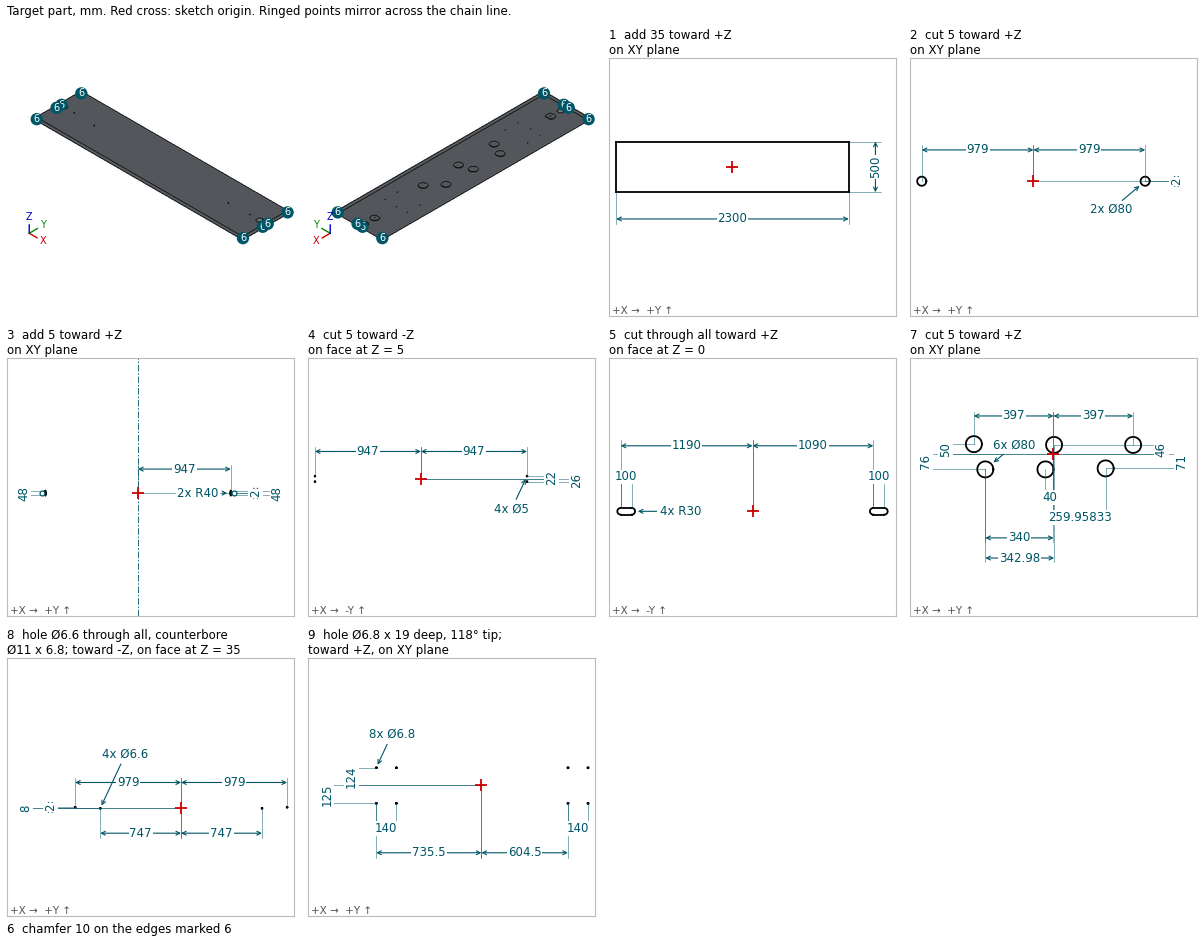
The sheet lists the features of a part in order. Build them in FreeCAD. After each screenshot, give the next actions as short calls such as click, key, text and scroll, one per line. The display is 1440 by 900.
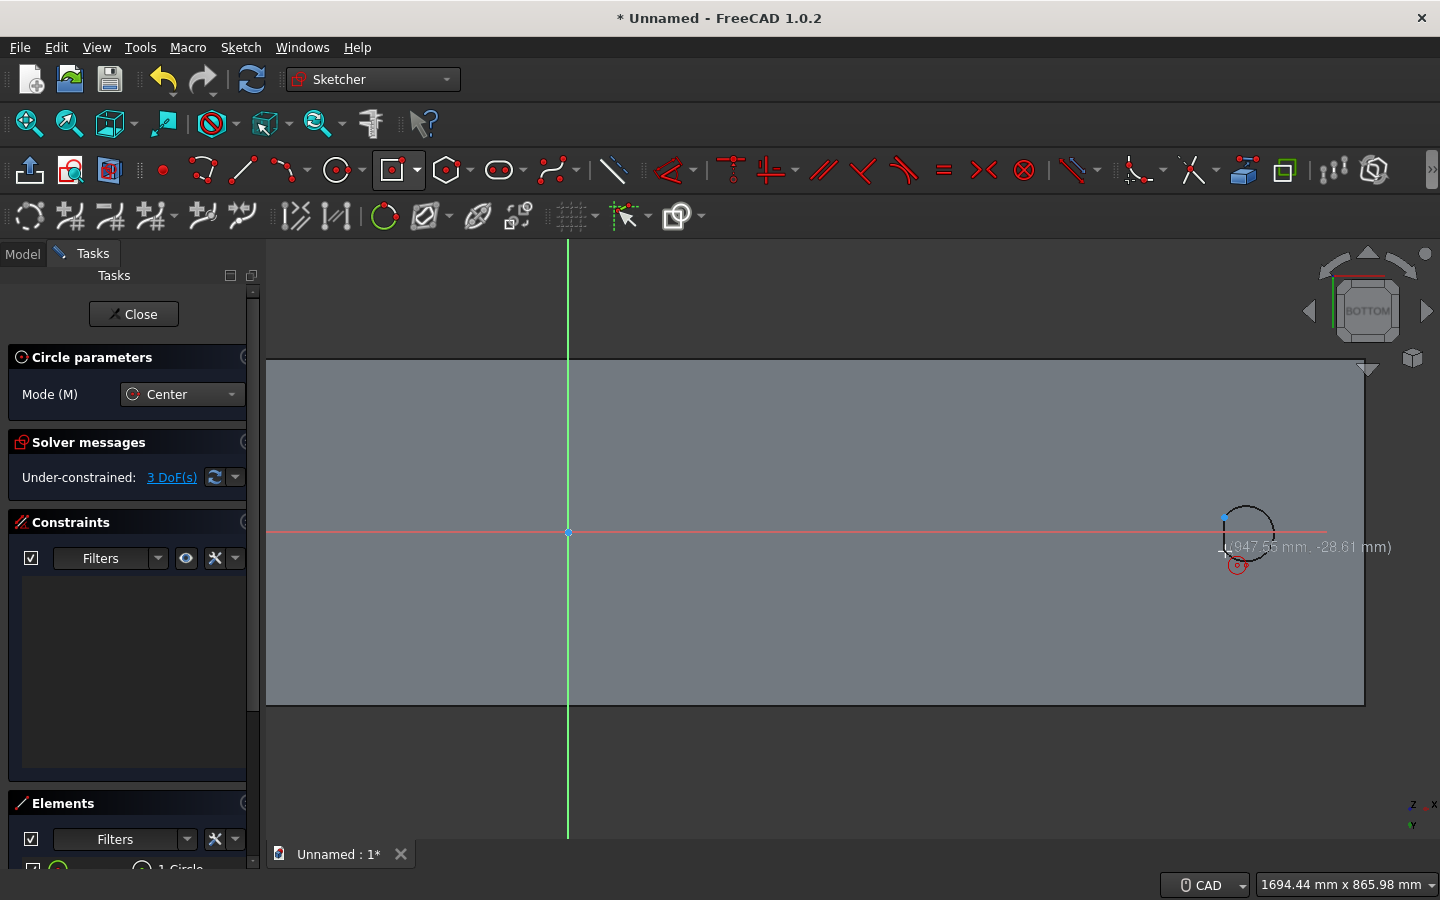
click(1224, 550)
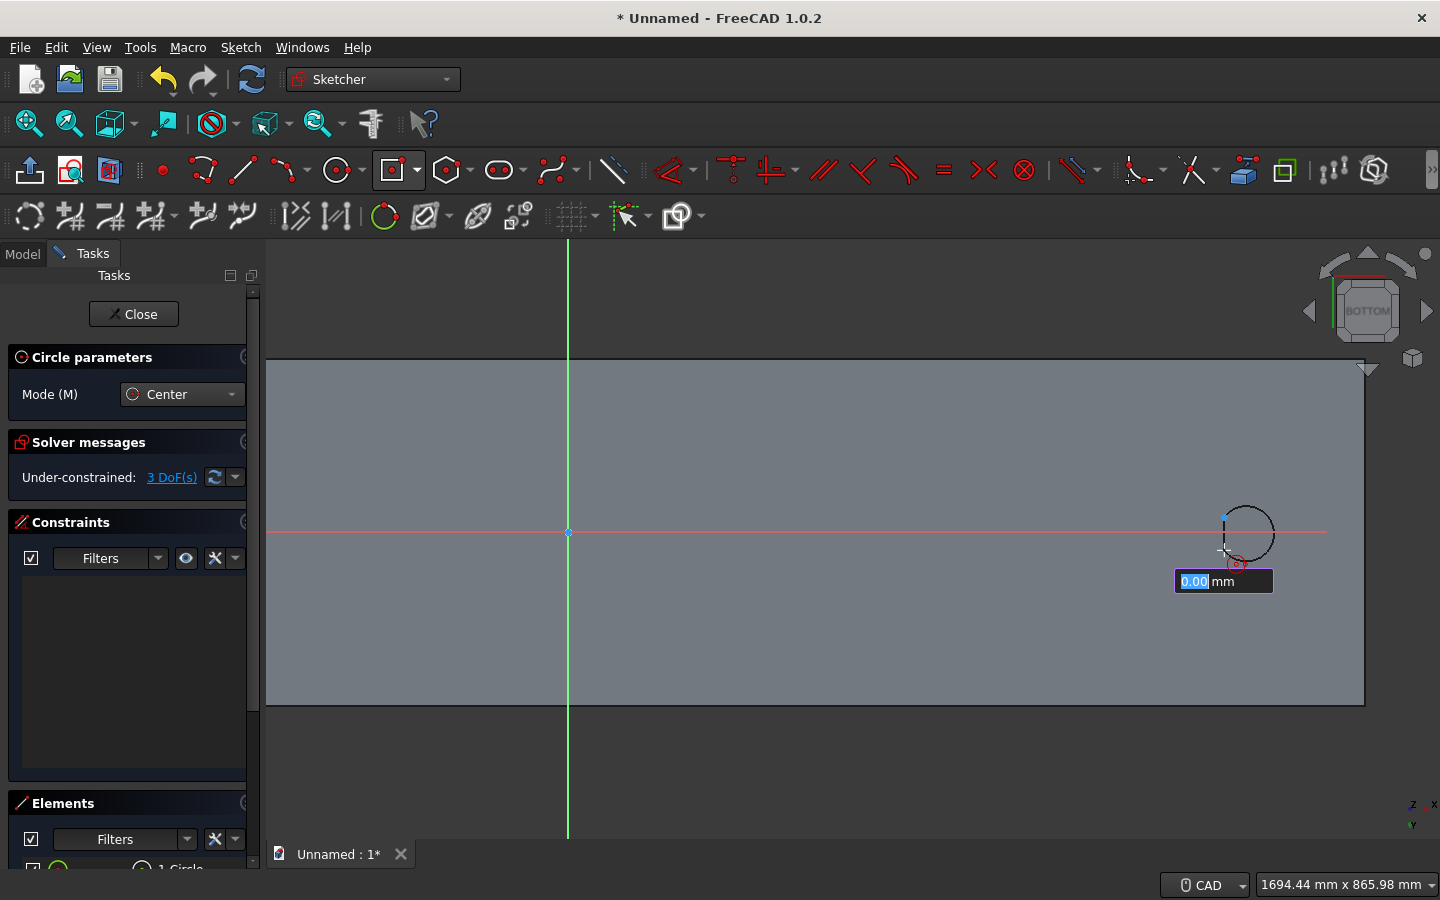
scroll(1225, 549, up, 12)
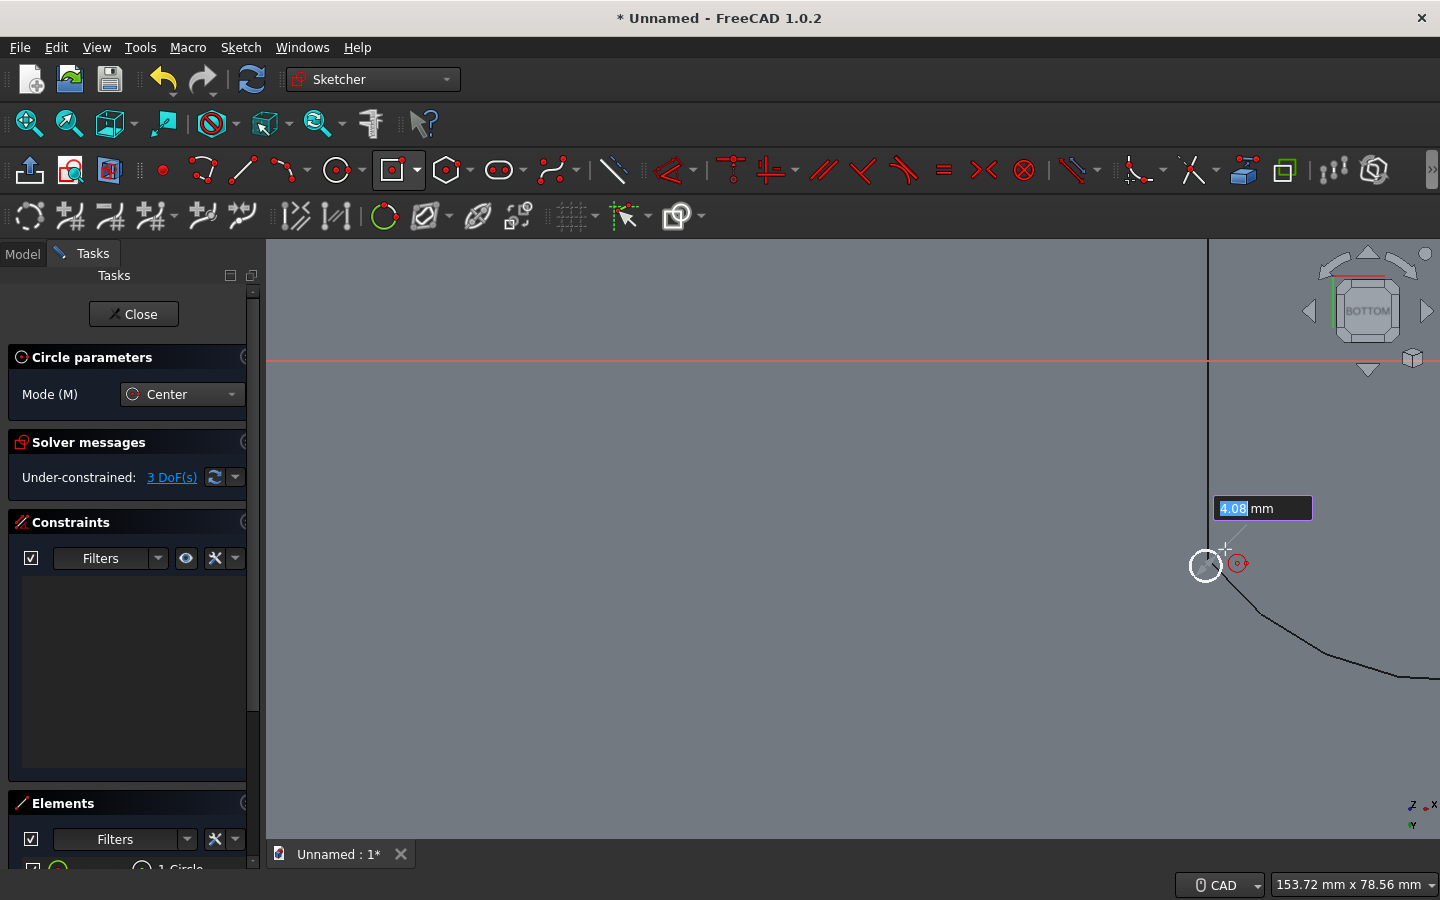
click(1222, 546)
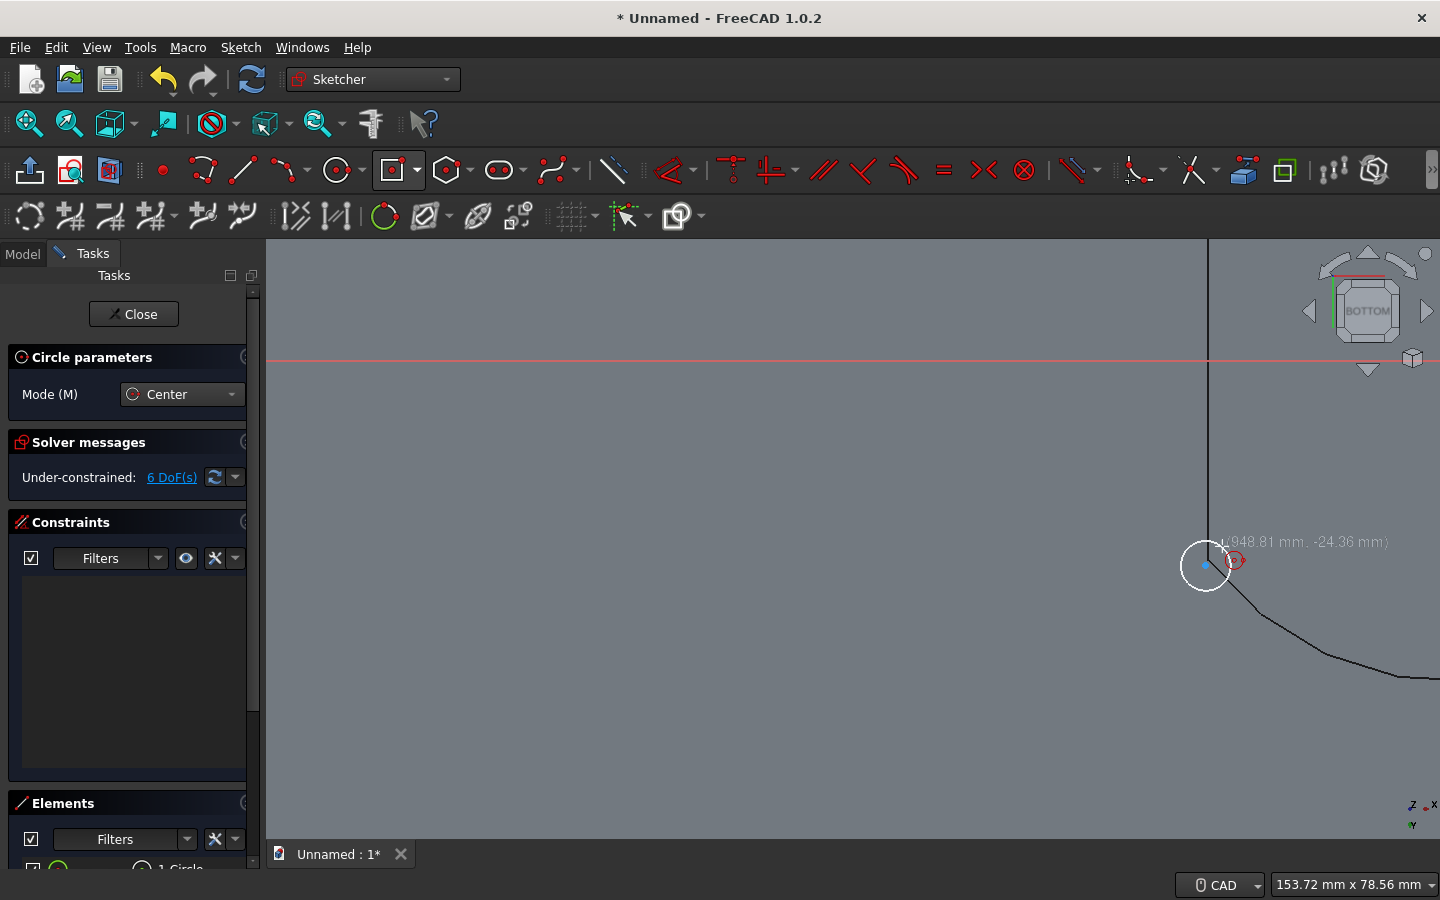
scroll(1141, 548, down, 15)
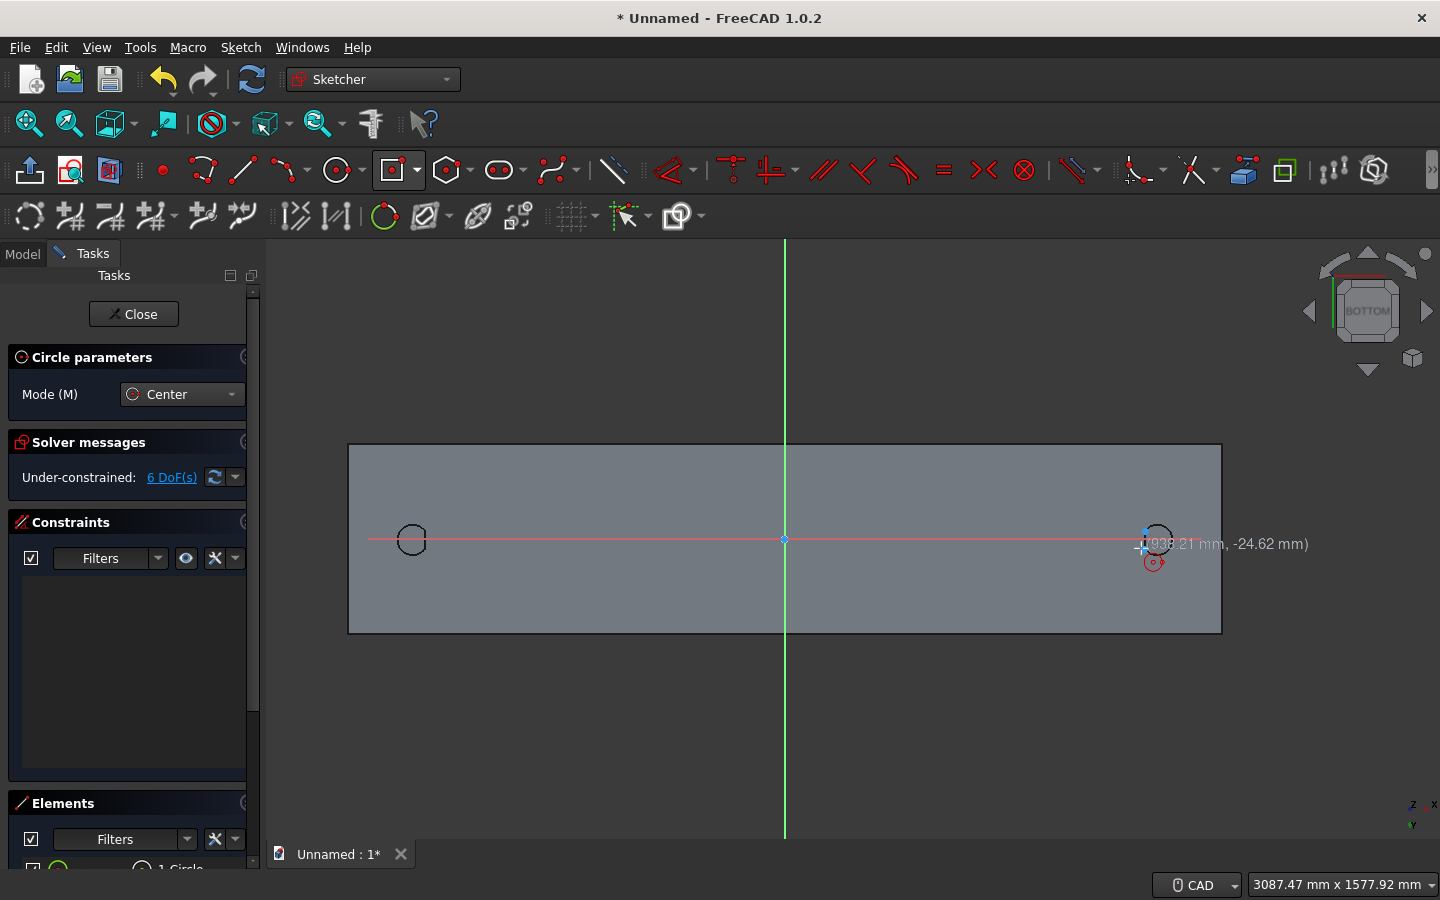
scroll(425, 531, up, 16)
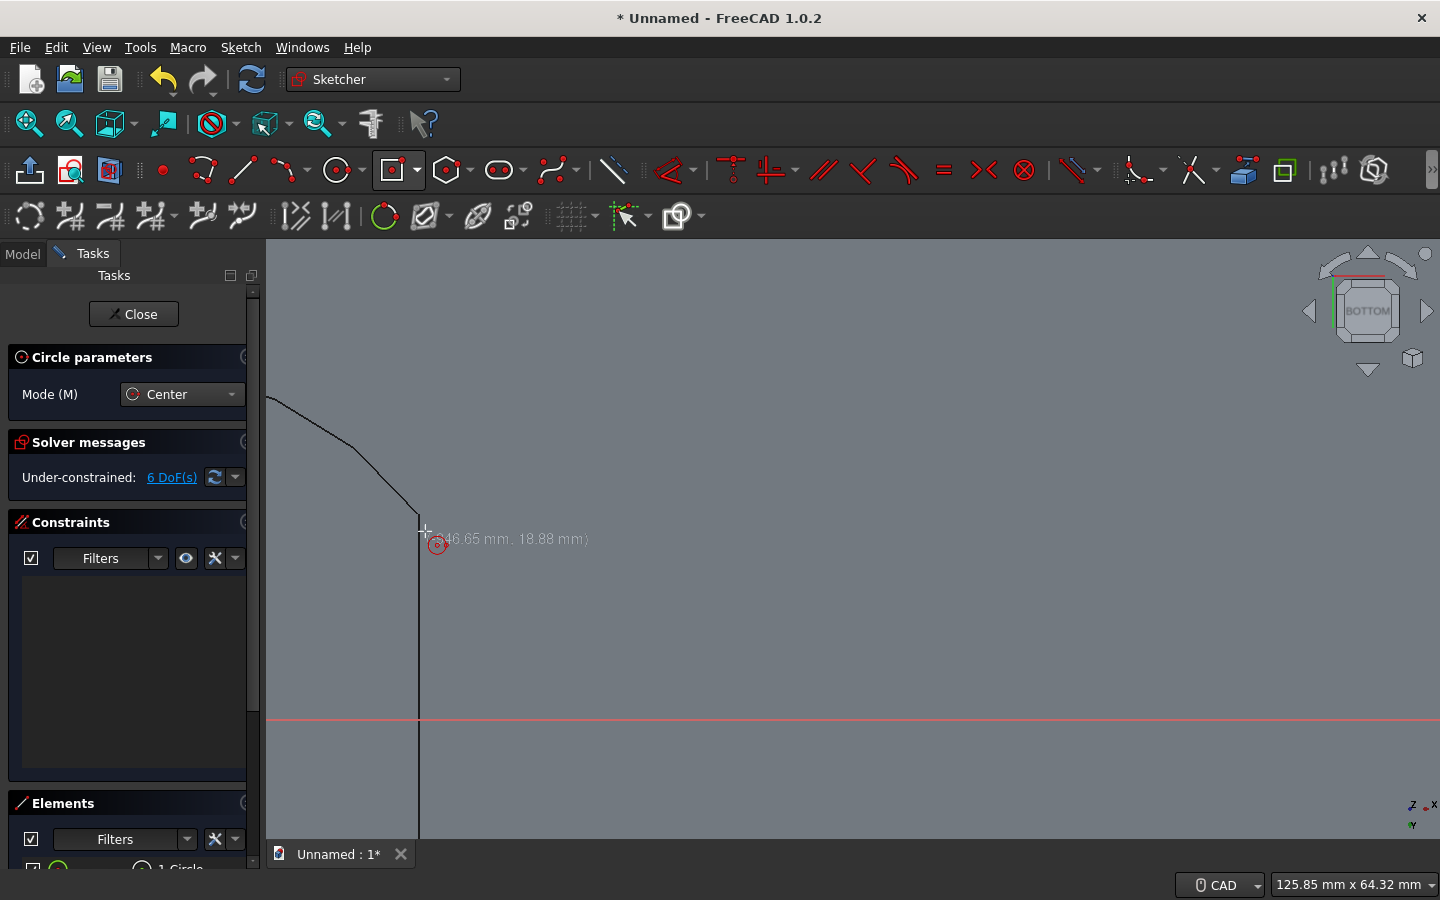
scroll(341, 529, down, 15)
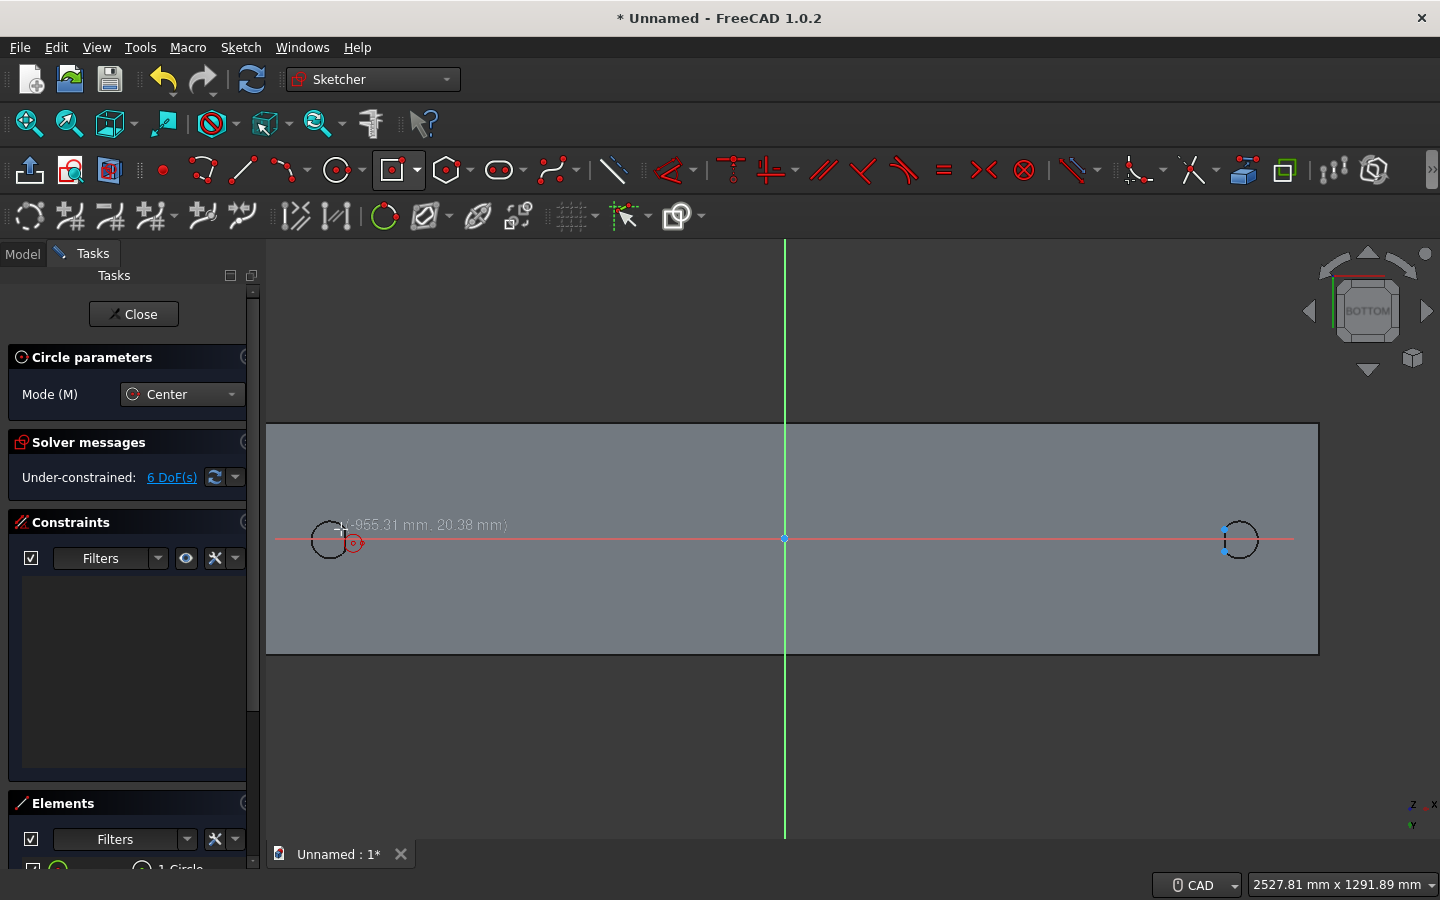
scroll(345, 529, up, 3)